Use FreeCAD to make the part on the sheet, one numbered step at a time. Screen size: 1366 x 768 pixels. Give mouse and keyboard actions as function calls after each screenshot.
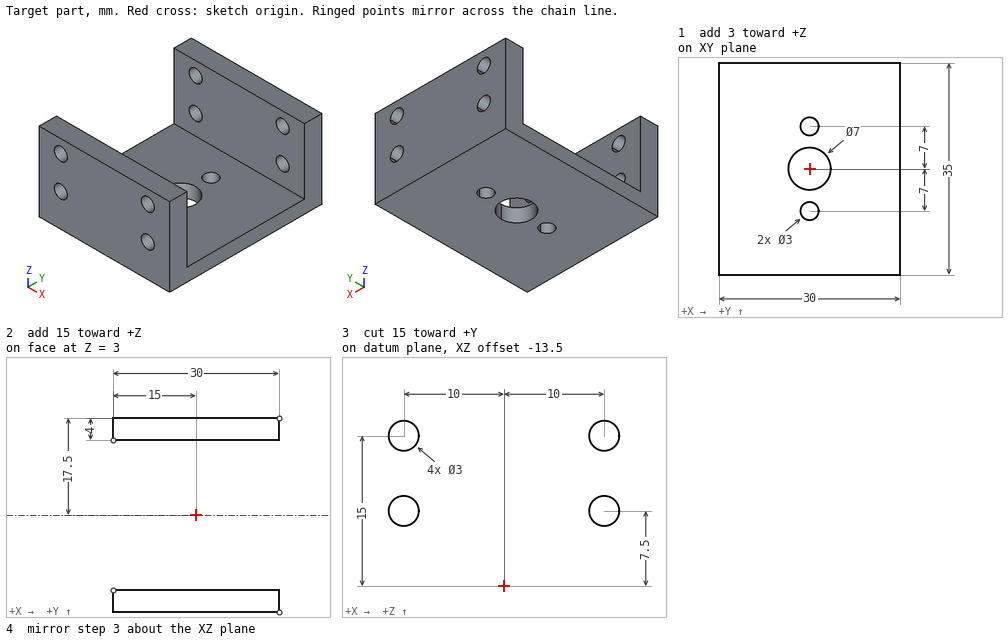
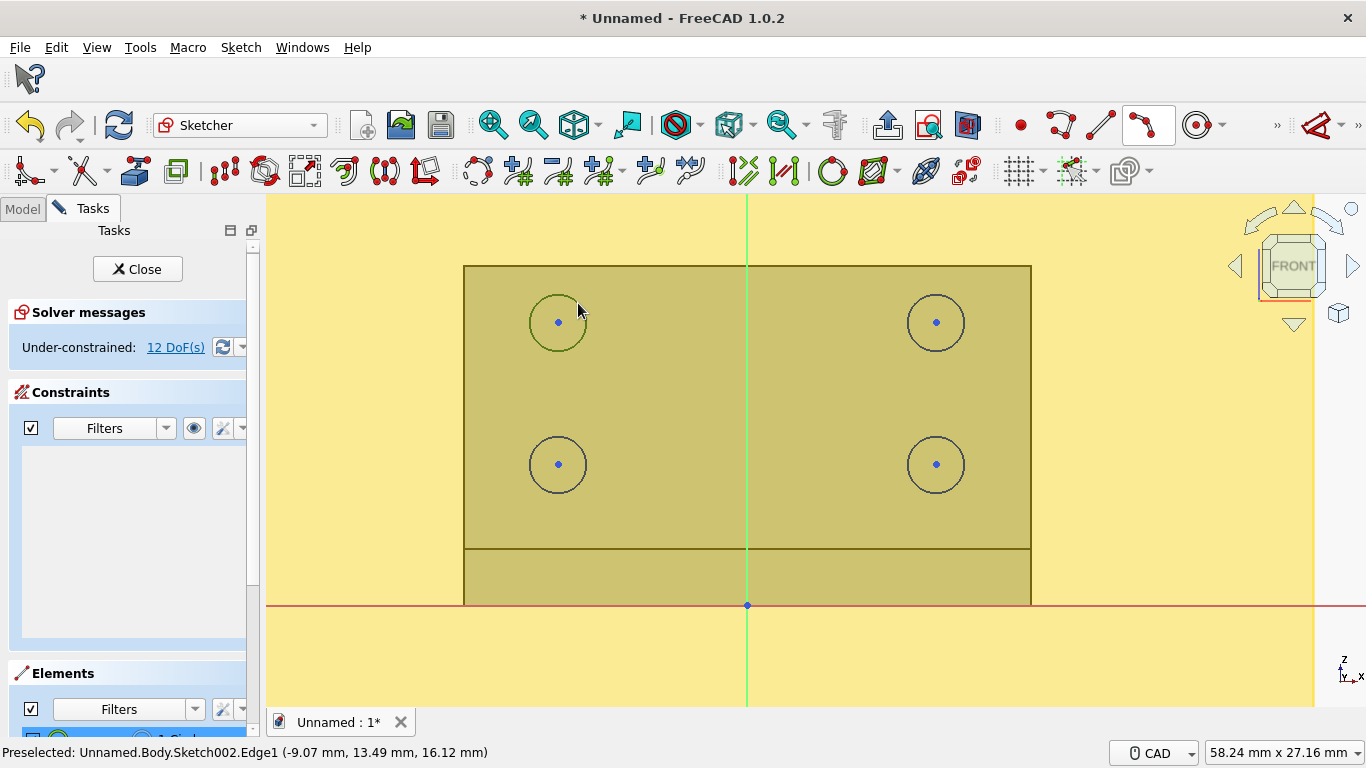
click(956, 303)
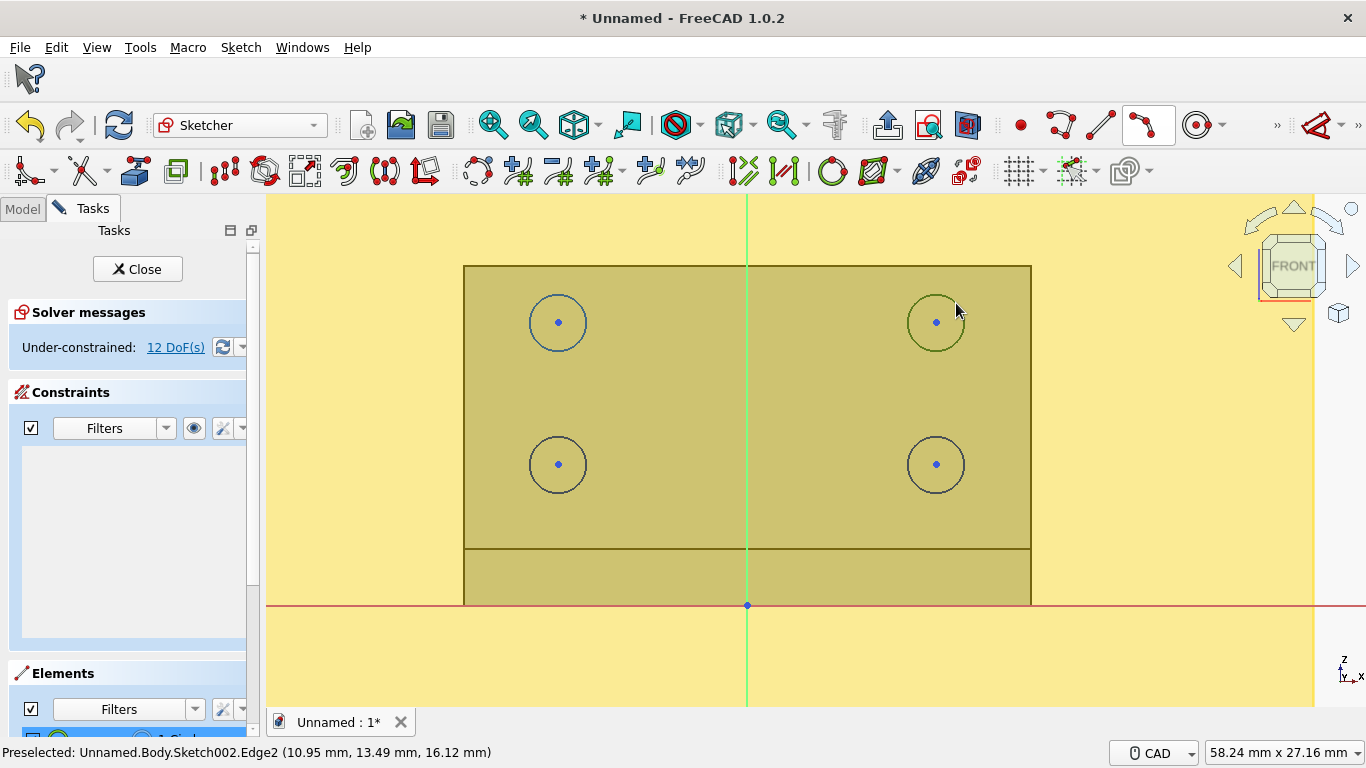
click(956, 445)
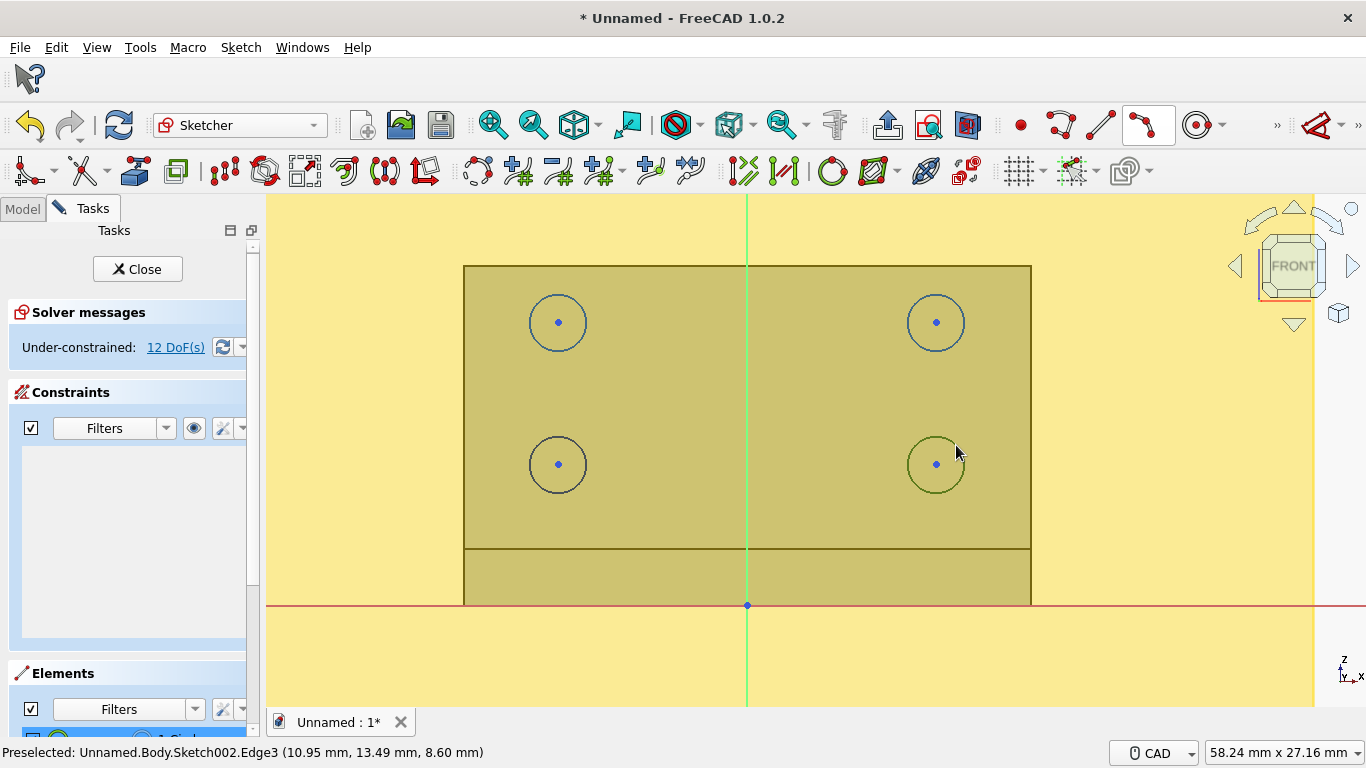
click(578, 445)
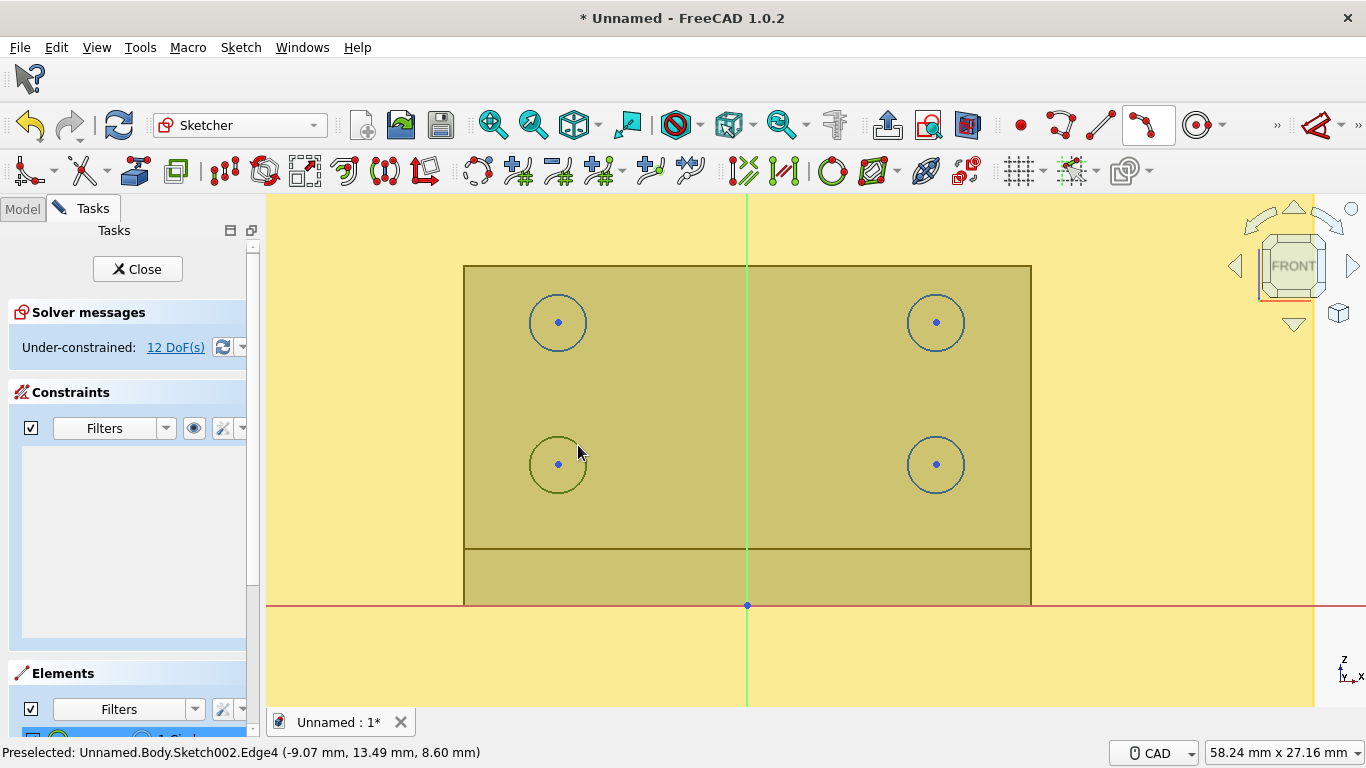
key(e)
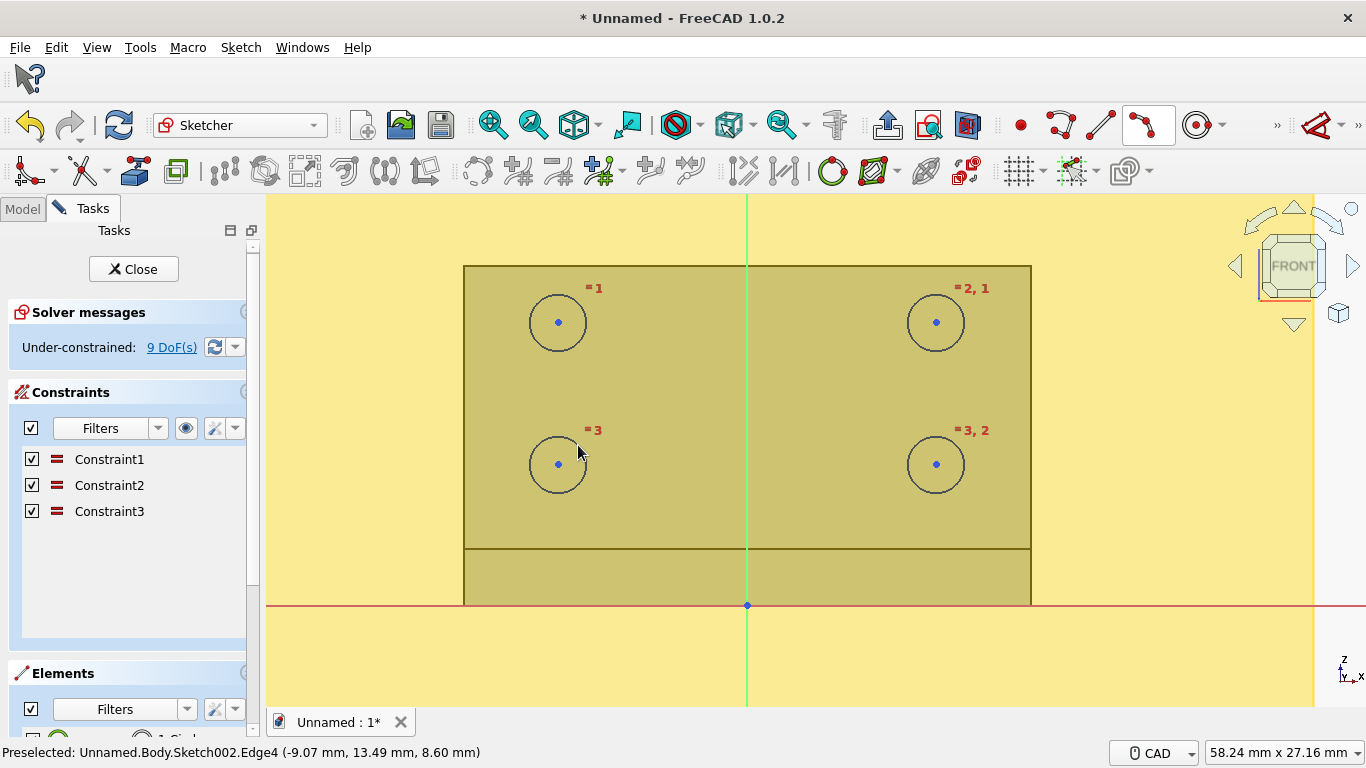
click(558, 323)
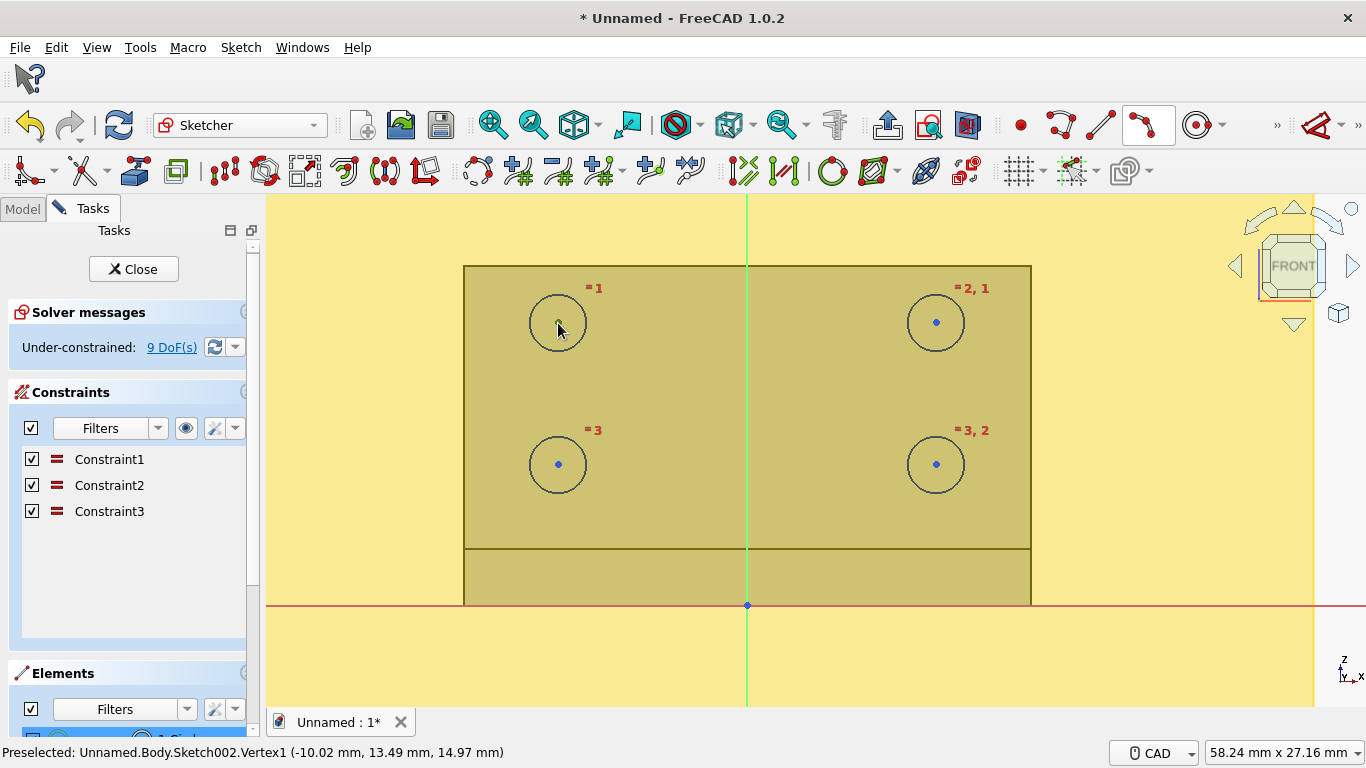
click(936, 323)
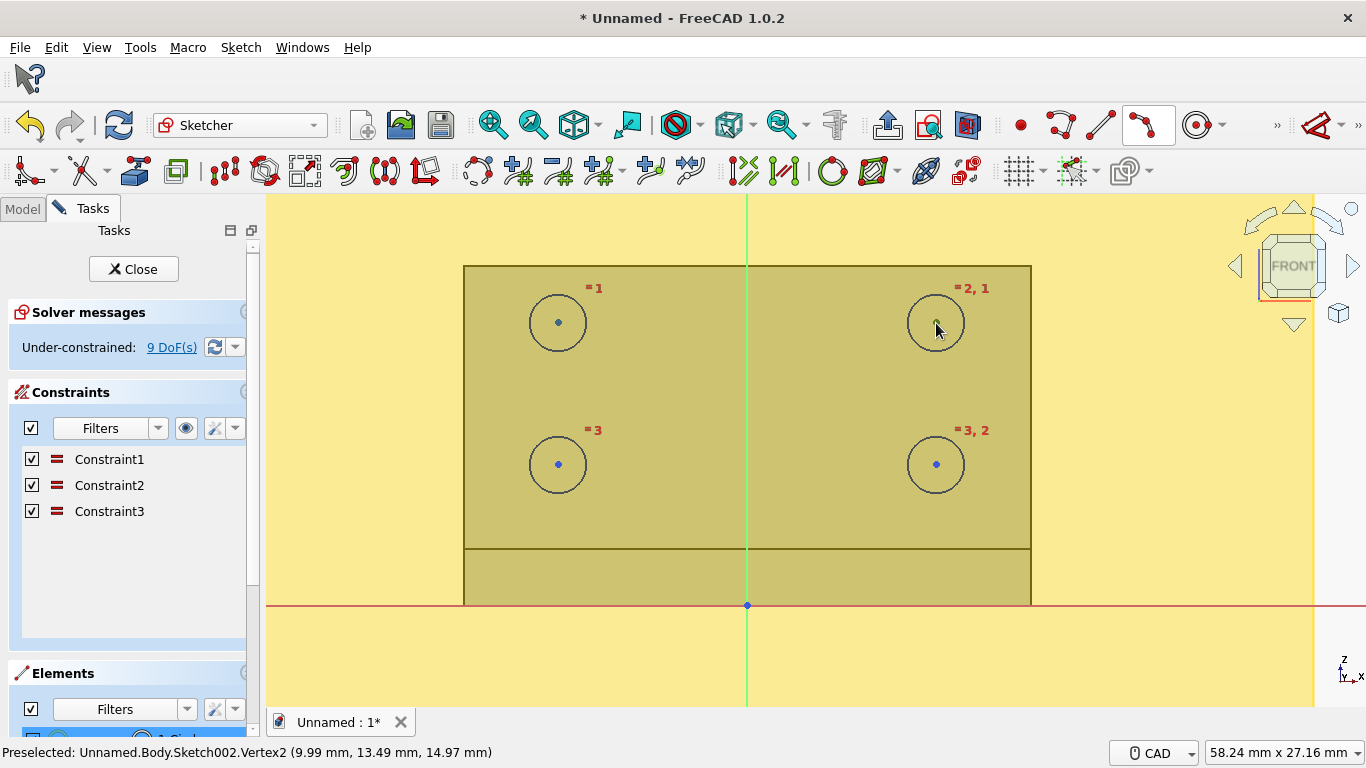
key(h)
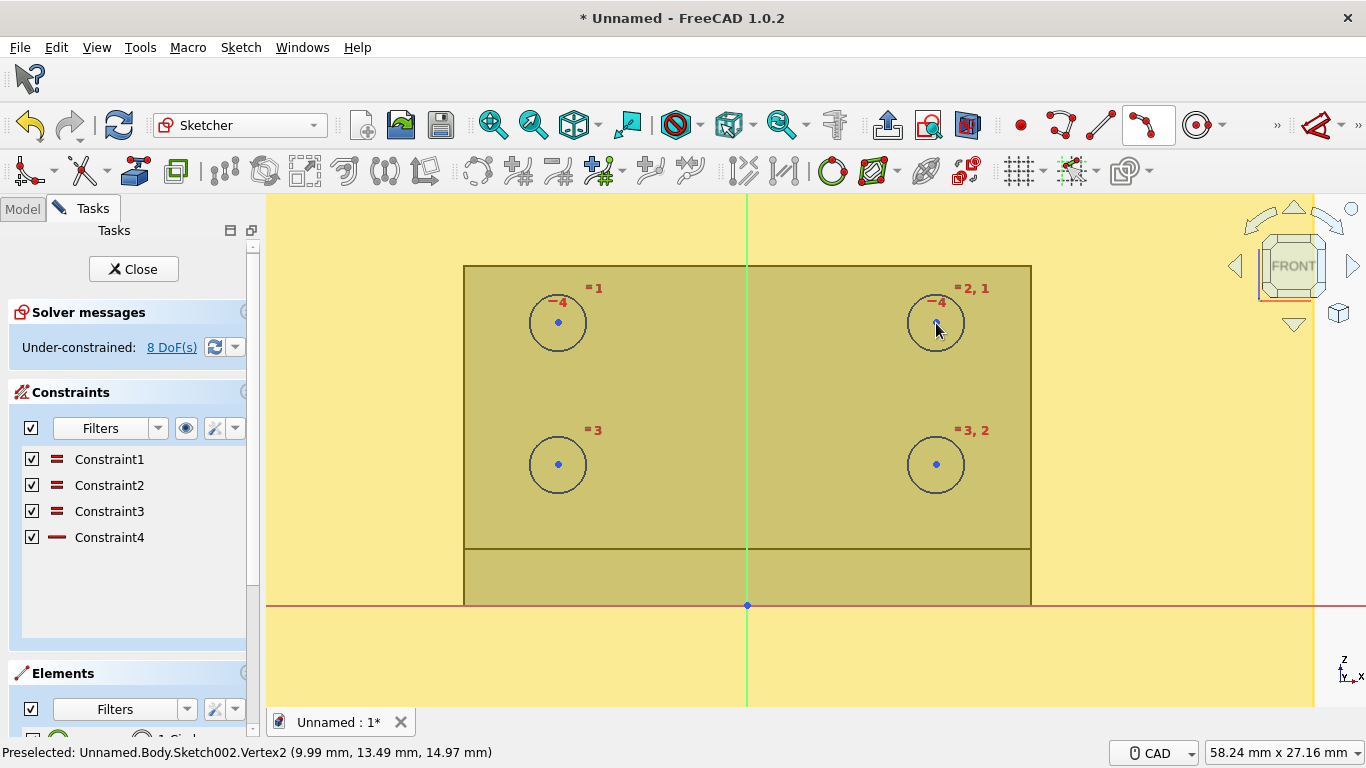
click(936, 323)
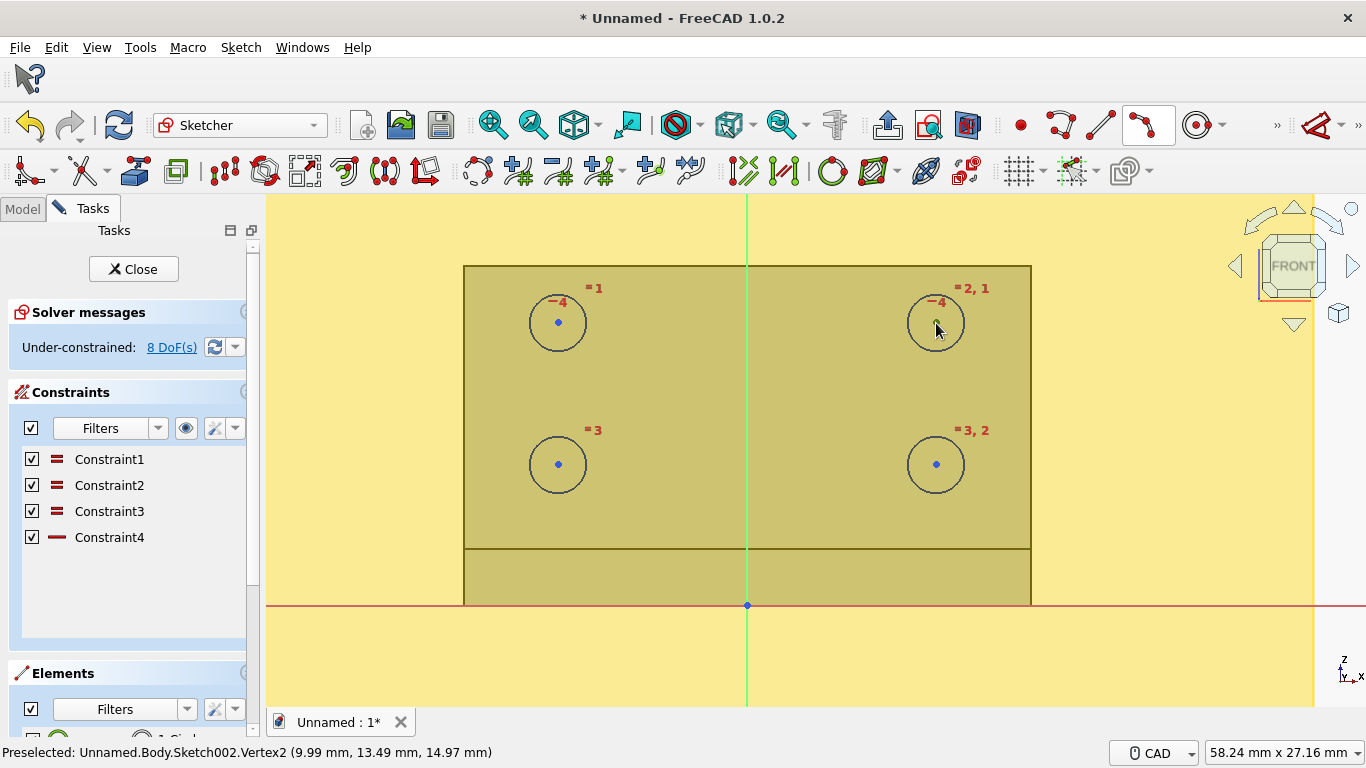
click(936, 465)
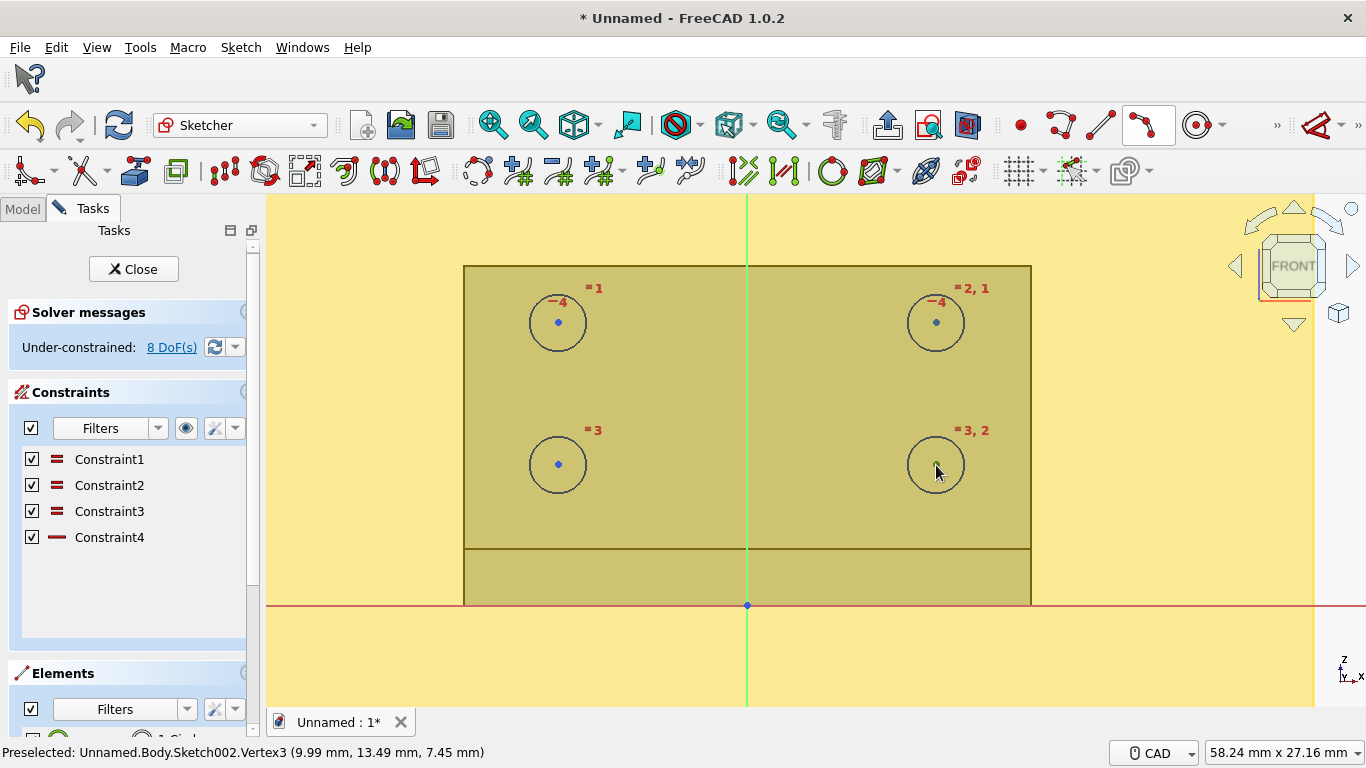
key(v)